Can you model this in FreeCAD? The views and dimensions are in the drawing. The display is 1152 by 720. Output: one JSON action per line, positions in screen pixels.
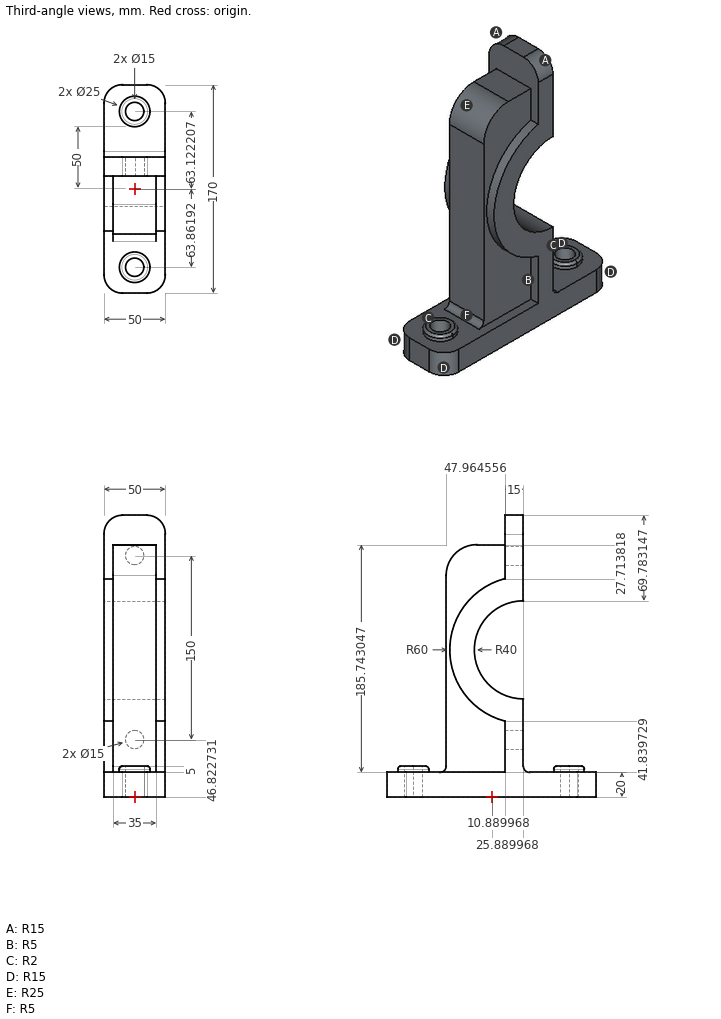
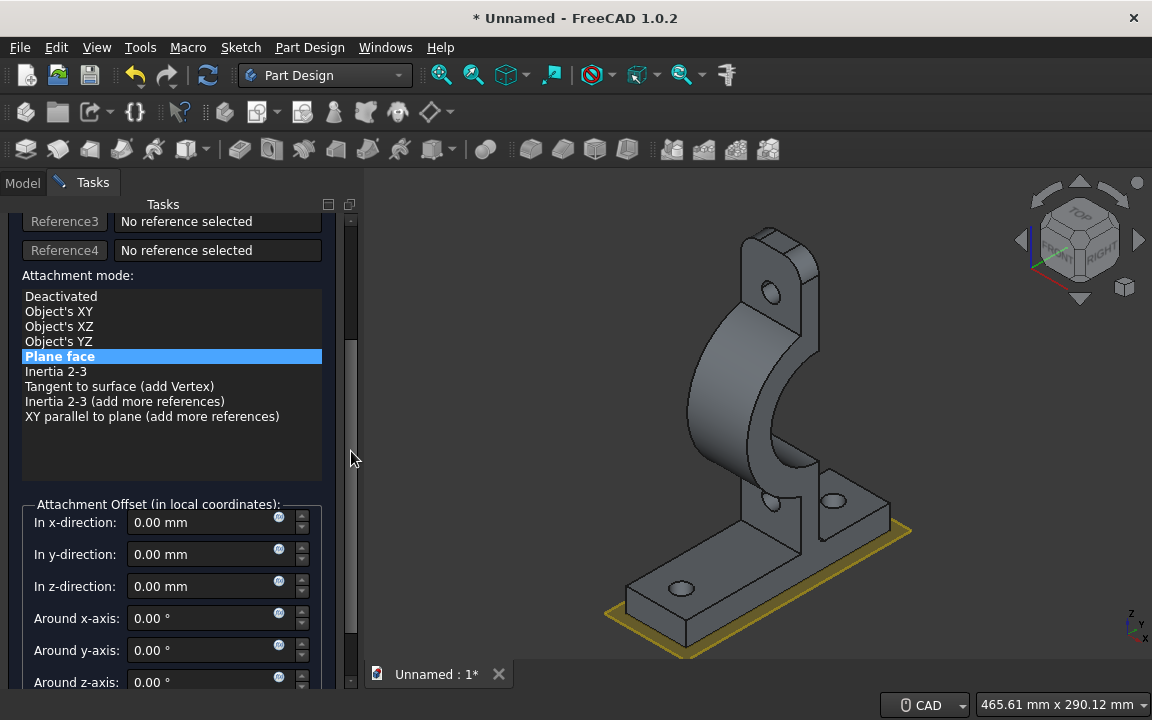
{"action": "triple_click", "coordinate": [210, 586]}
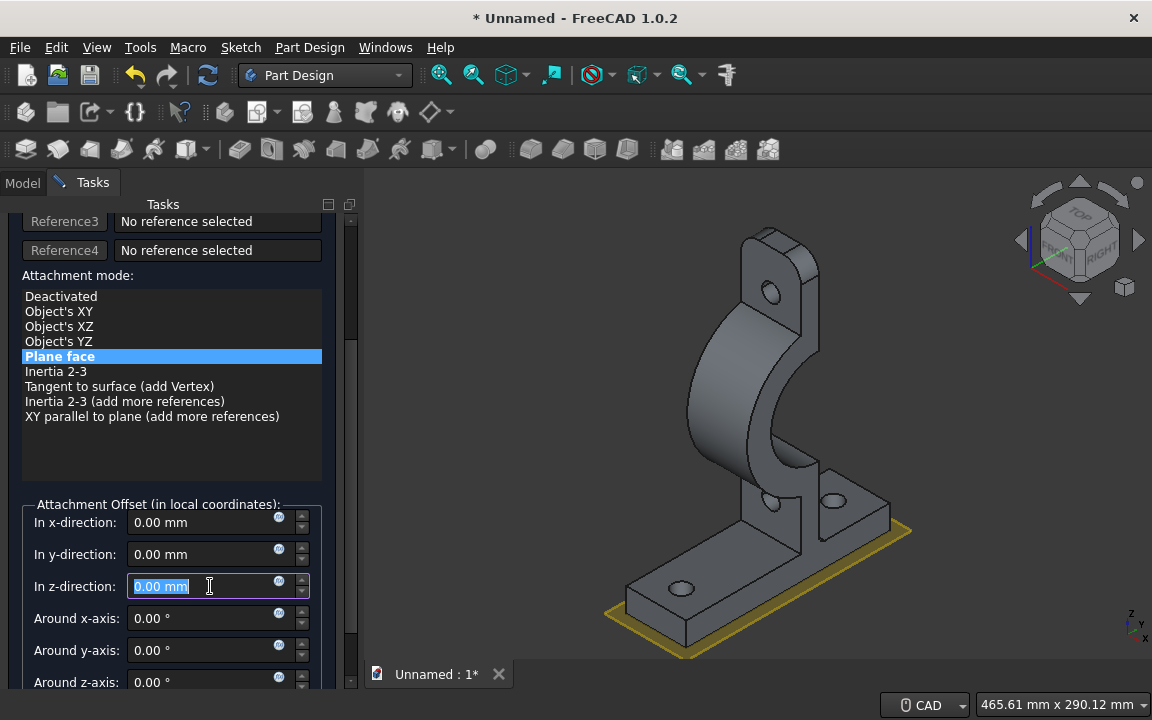
{"action": "type", "text": "25"}
{"action": "key", "text": "Tab"}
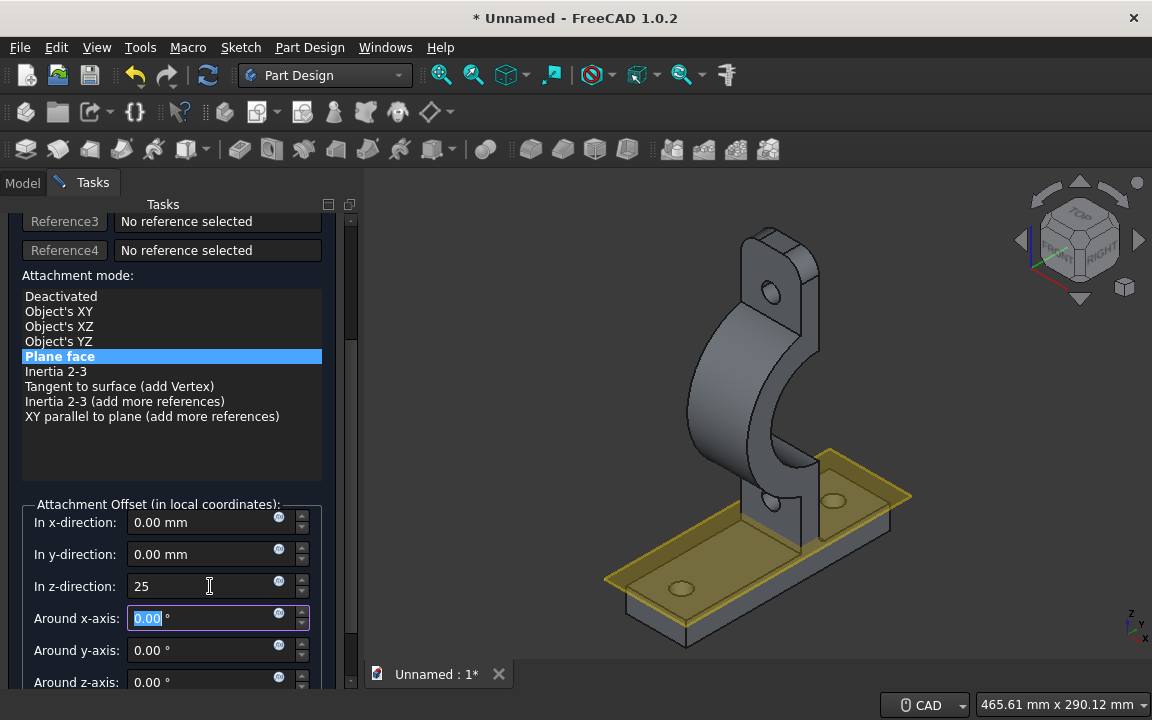
{"action": "scroll", "coordinate": [351, 451], "scroll_direction": "up", "scroll_amount": 4}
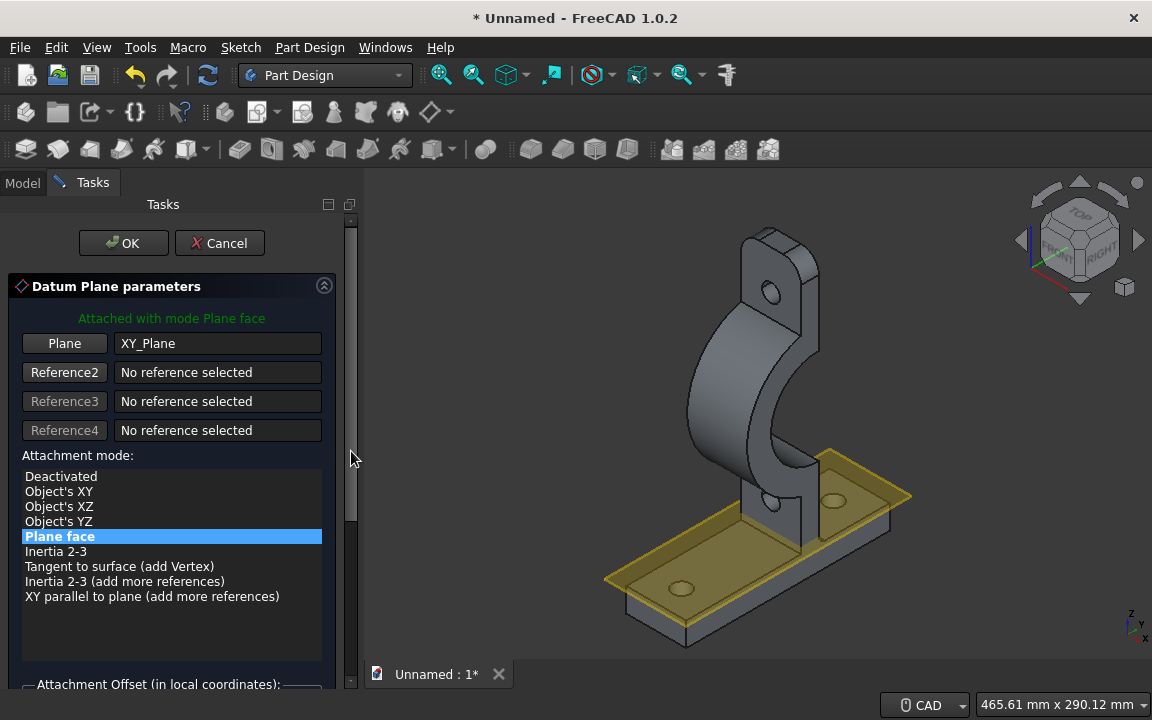
{"action": "left_click", "coordinate": [124, 243]}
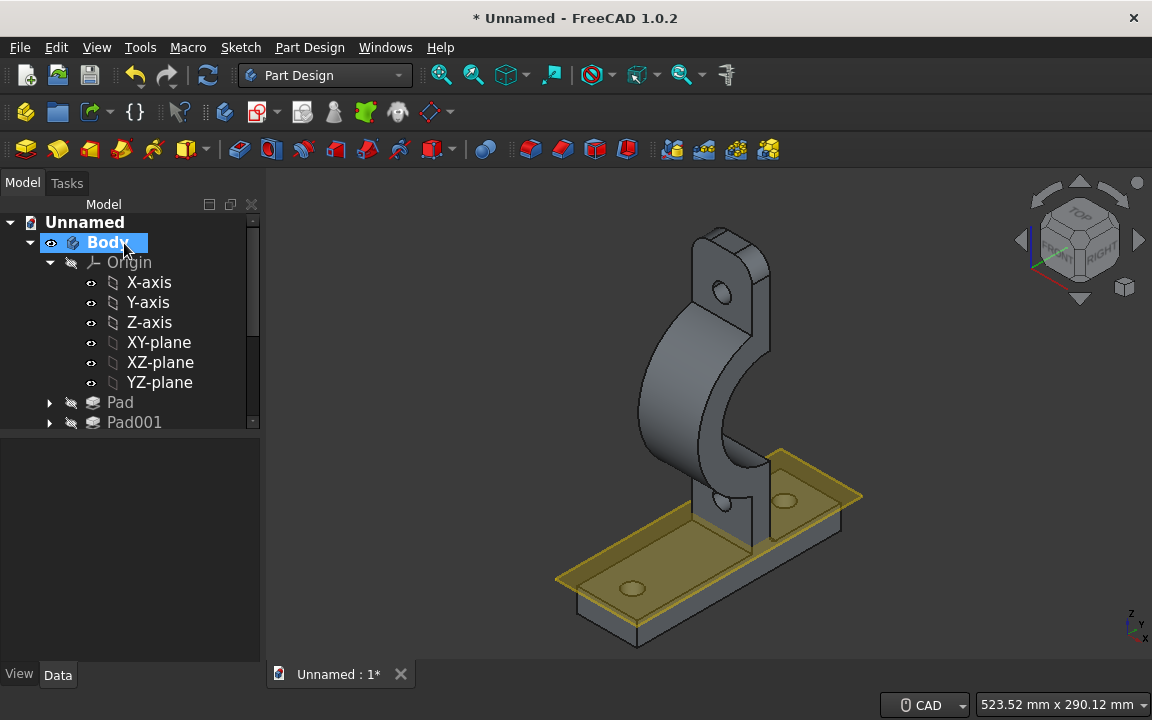
{"action": "scroll", "coordinate": [100, 318], "scroll_direction": "down", "scroll_amount": 3}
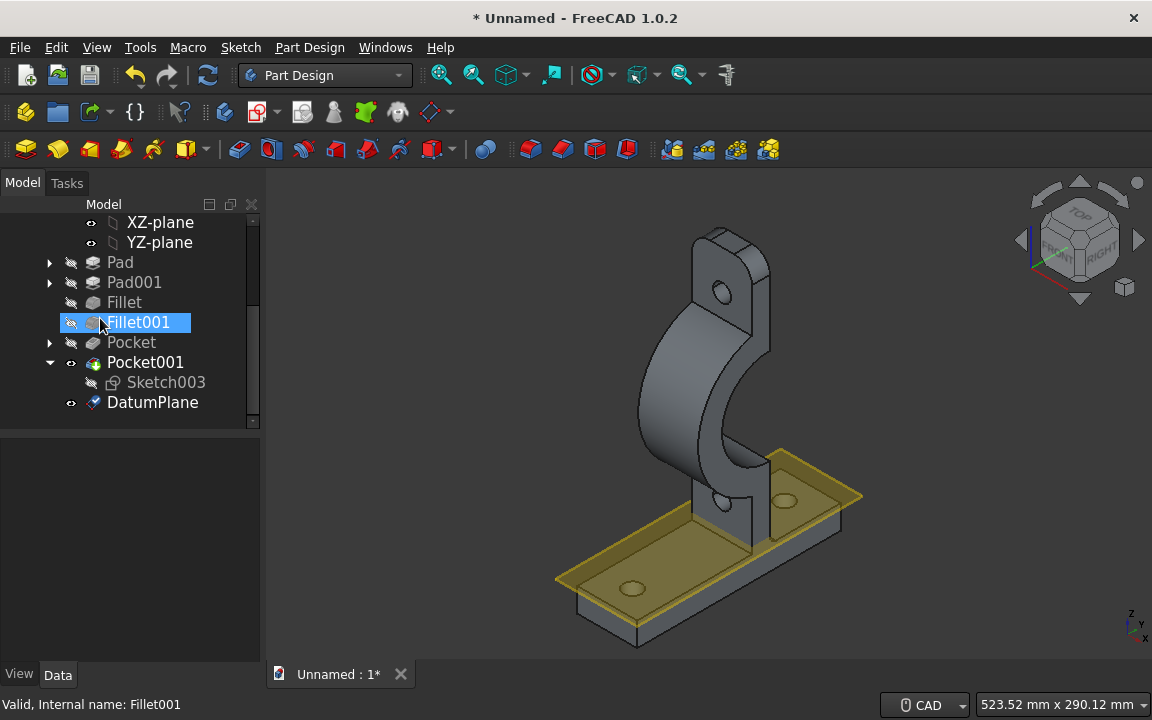
{"action": "left_click", "coordinate": [116, 403]}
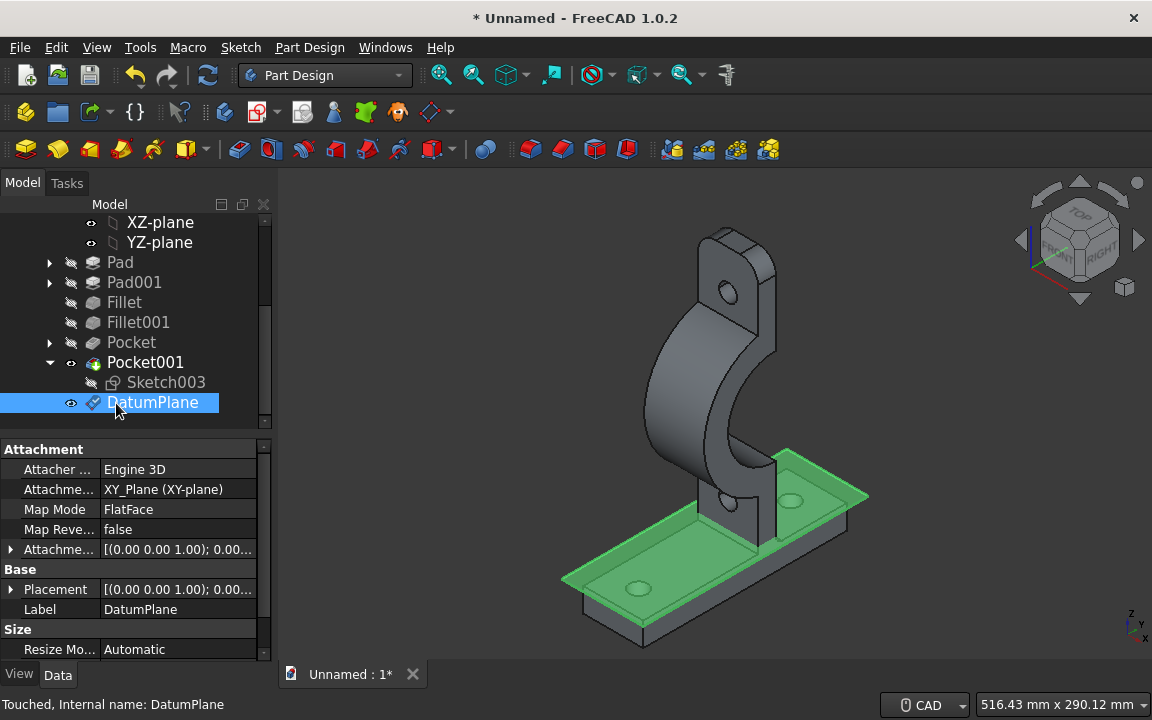
{"action": "left_click", "coordinate": [258, 112]}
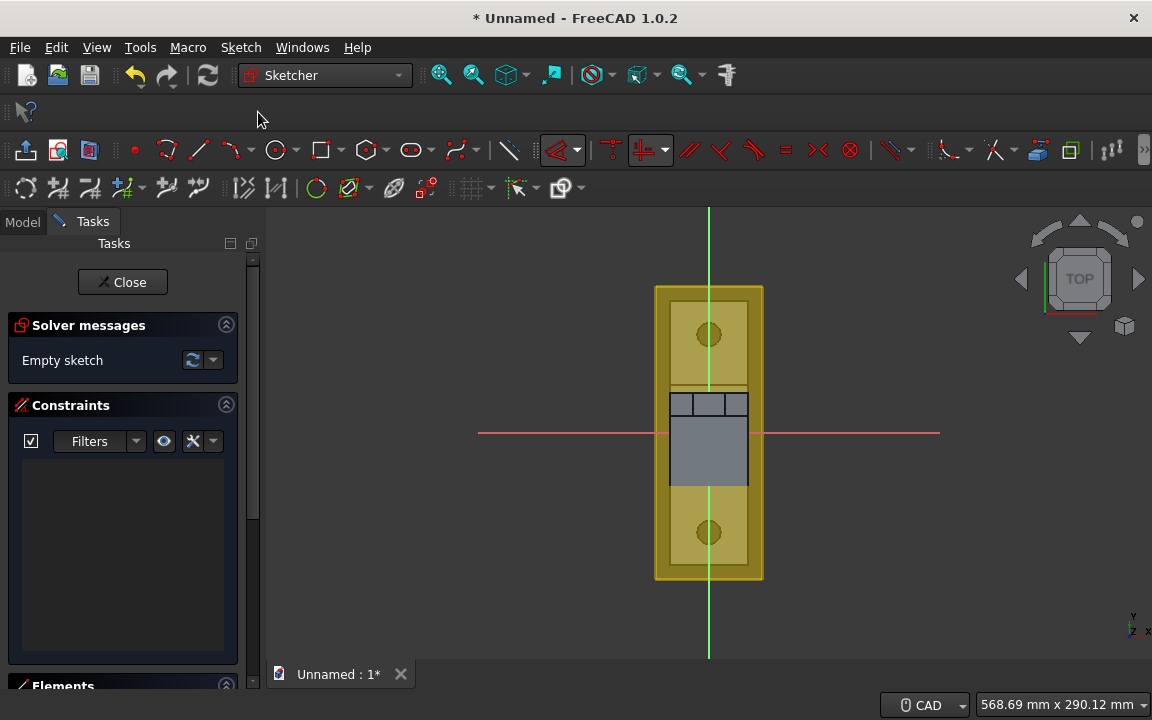
{"action": "key", "text": "q s"}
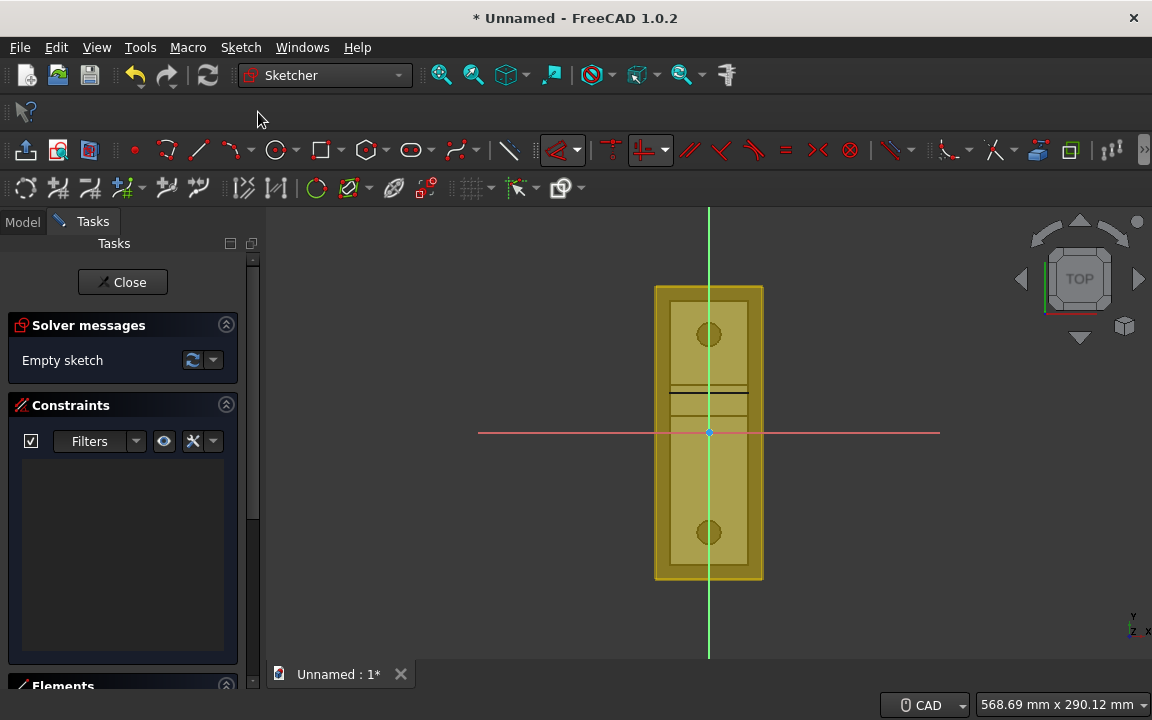
{"action": "key", "text": "g c"}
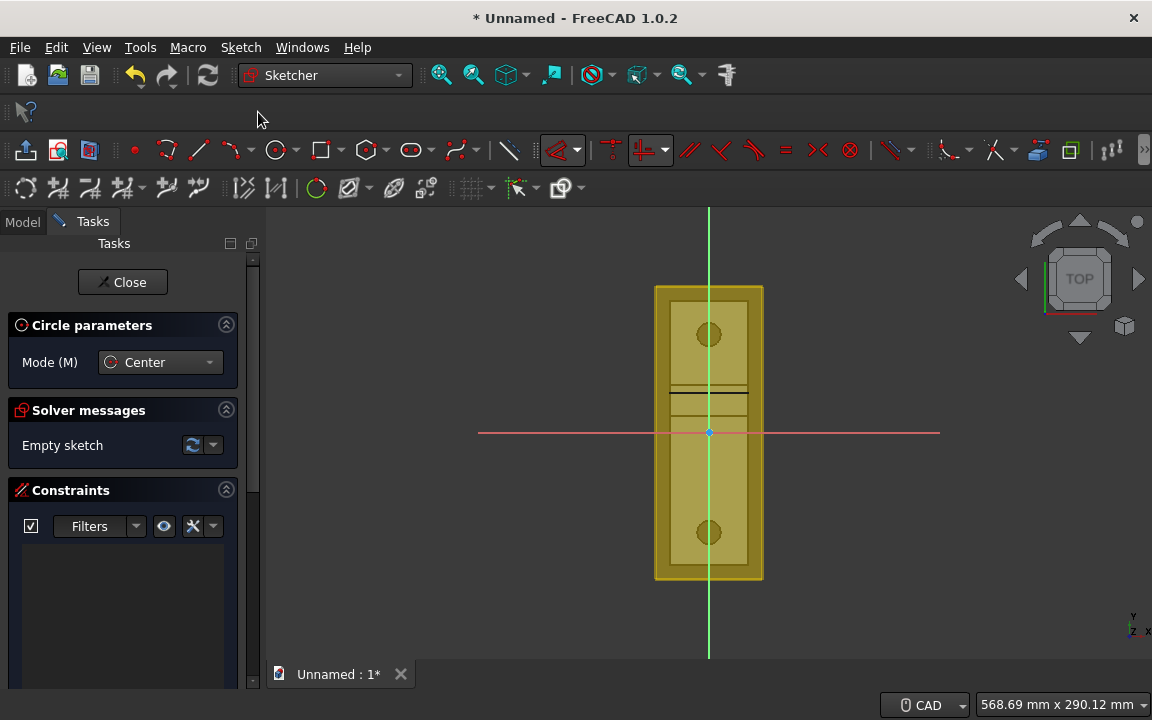
{"action": "left_click", "coordinate": [709, 335]}
{"action": "mouse_move", "coordinate": [727, 328]}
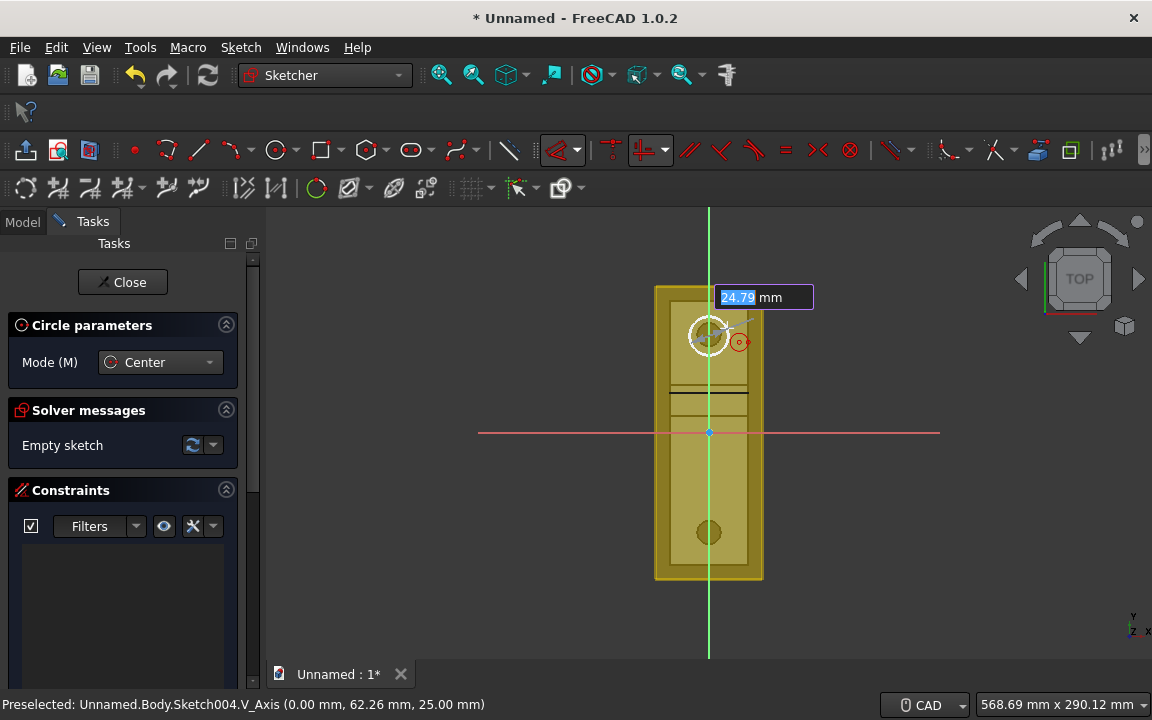
{"action": "type", "text": "25"}
{"action": "key", "text": "Return"}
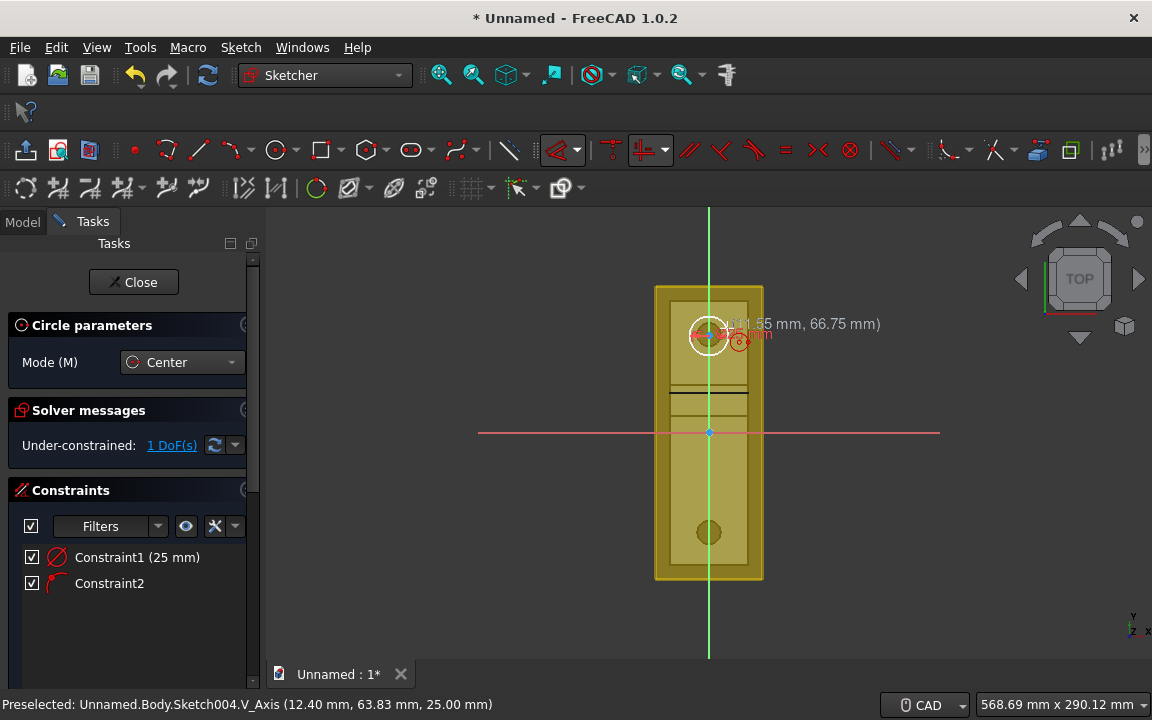
{"action": "left_click", "coordinate": [709, 532]}
{"action": "mouse_move", "coordinate": [727, 526]}